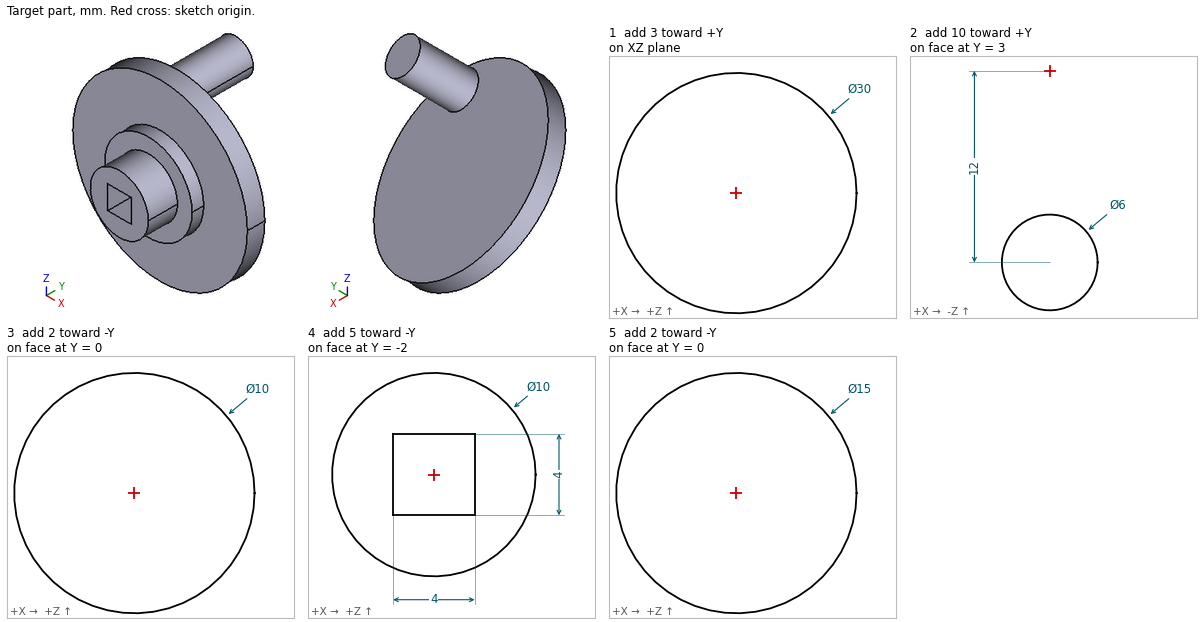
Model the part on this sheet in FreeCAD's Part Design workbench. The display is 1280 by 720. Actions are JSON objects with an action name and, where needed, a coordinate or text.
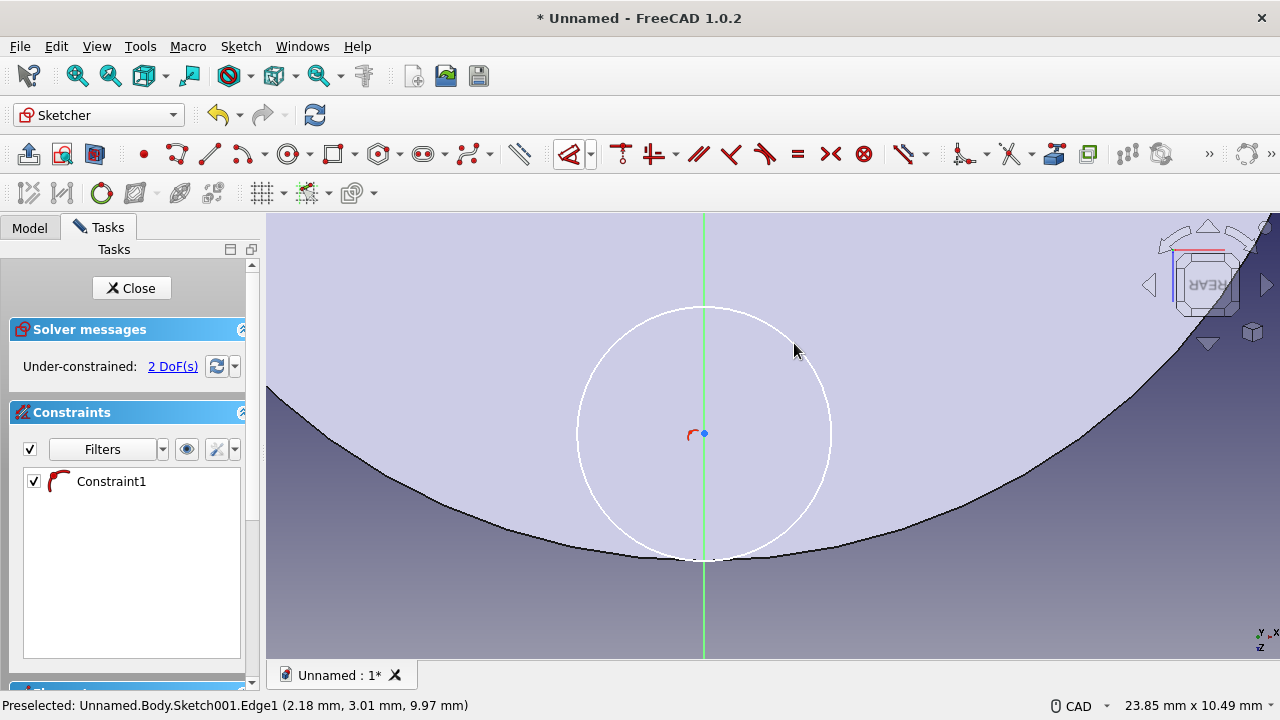
{"action": "left_click", "coordinate": [568, 154]}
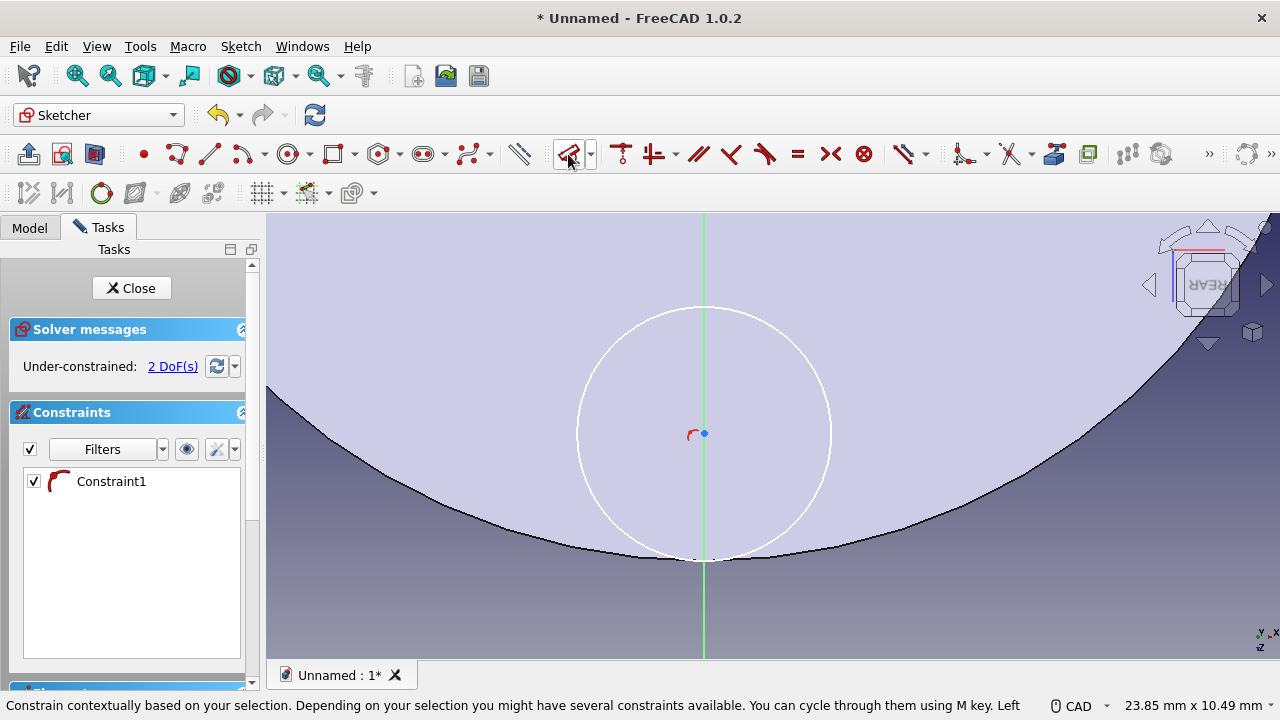
{"action": "left_click", "coordinate": [794, 344]}
{"action": "left_click", "coordinate": [817, 321]}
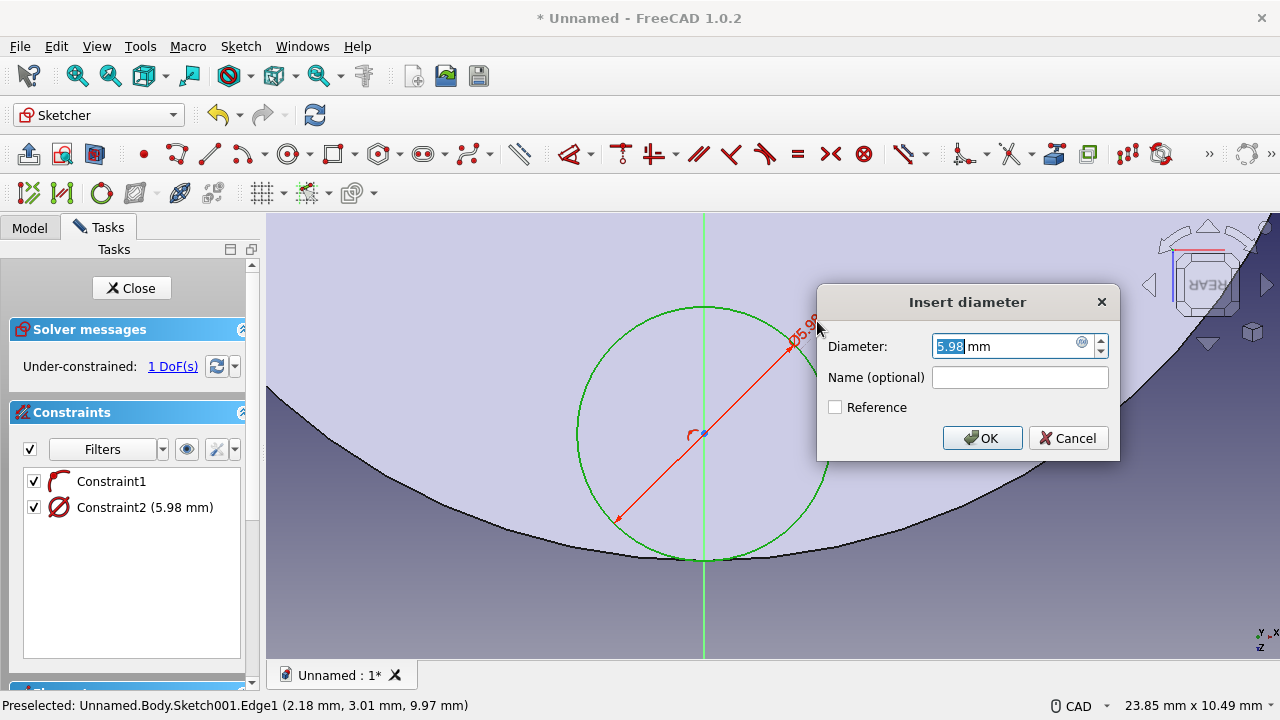
{"action": "type", "text": "6"}
{"action": "key", "text": "Return"}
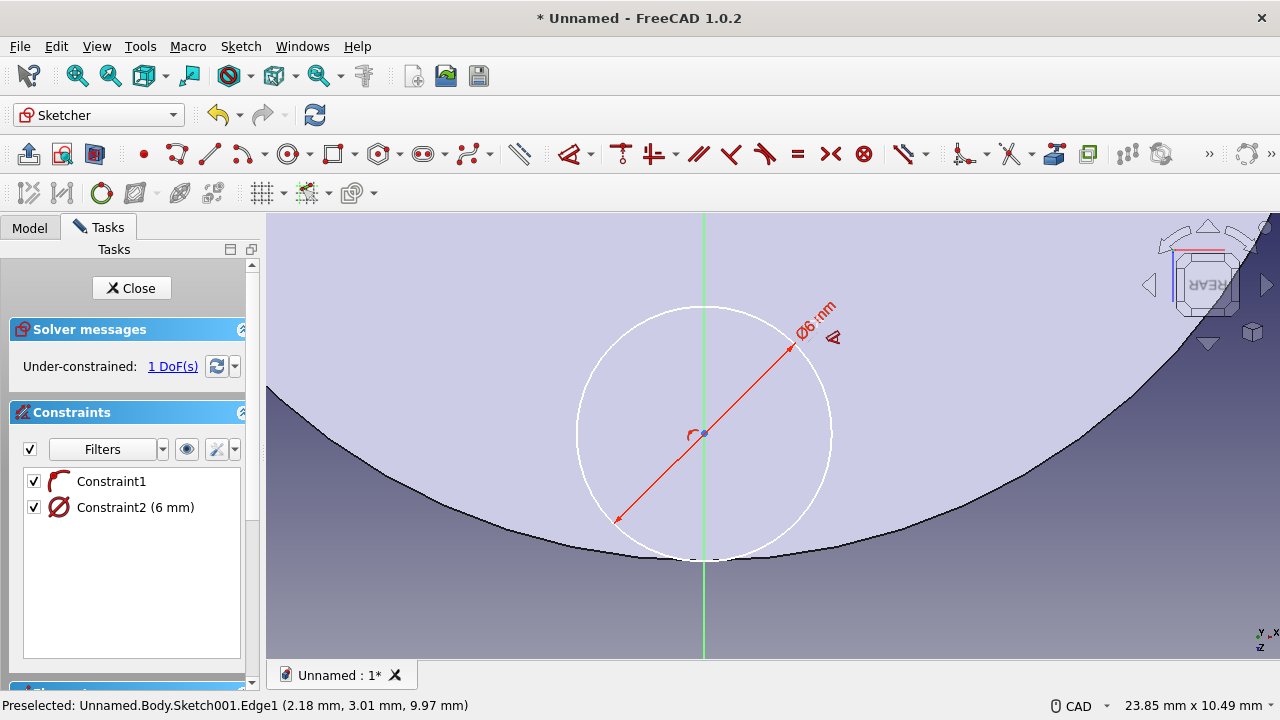
{"action": "left_click", "coordinate": [704, 434]}
{"action": "left_click", "coordinate": [738, 337]}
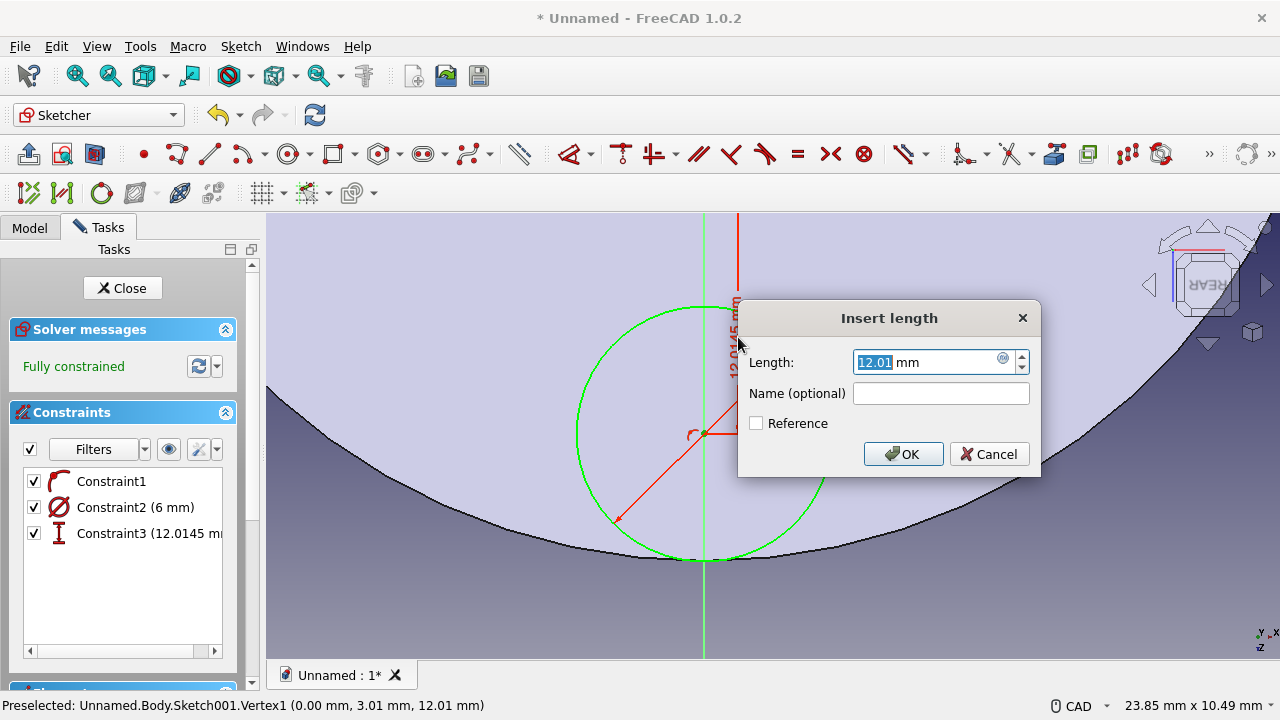
{"action": "type", "text": "12"}
{"action": "key", "text": "Return"}
{"action": "key", "text": "Escape"}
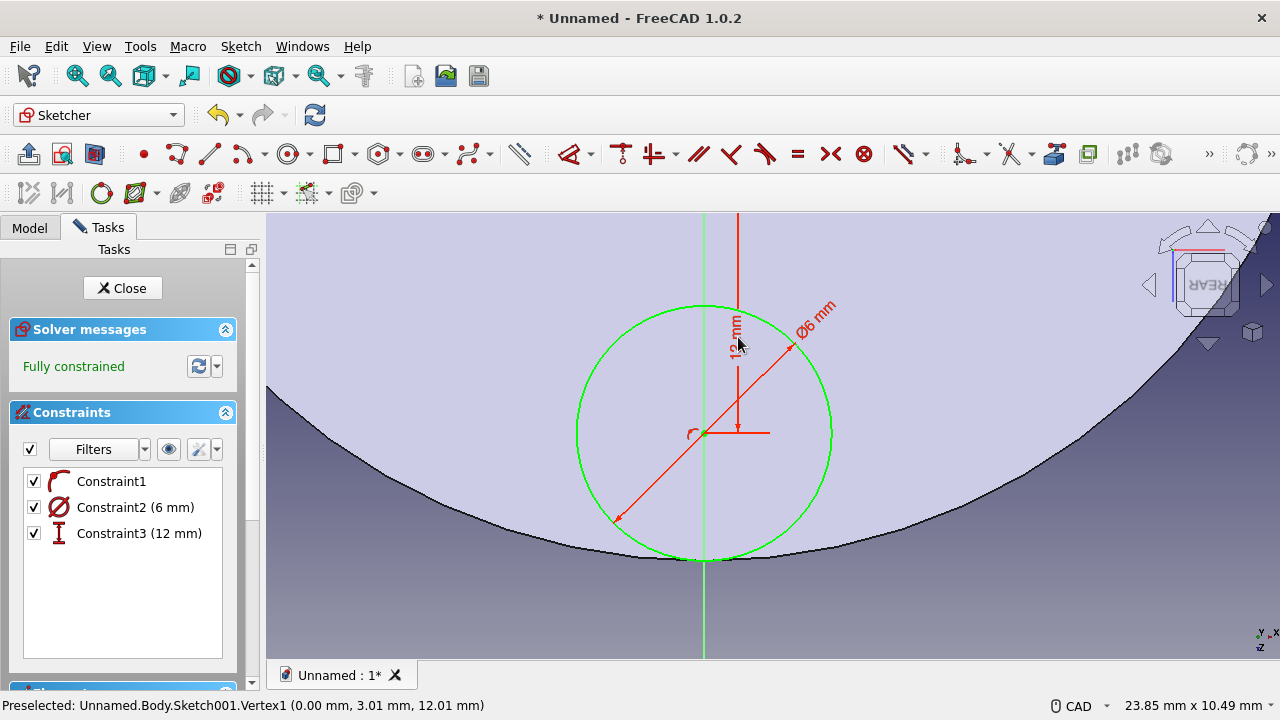
{"action": "left_click", "coordinate": [123, 288]}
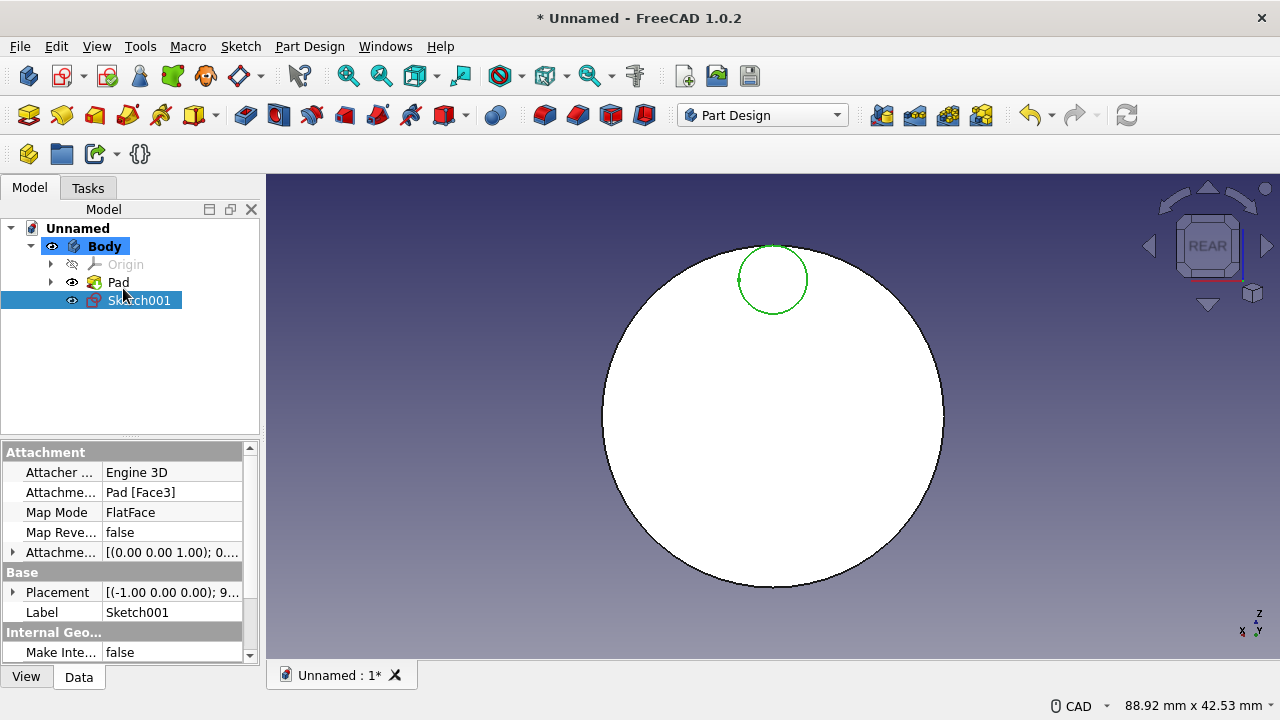
{"action": "left_click", "coordinate": [29, 116]}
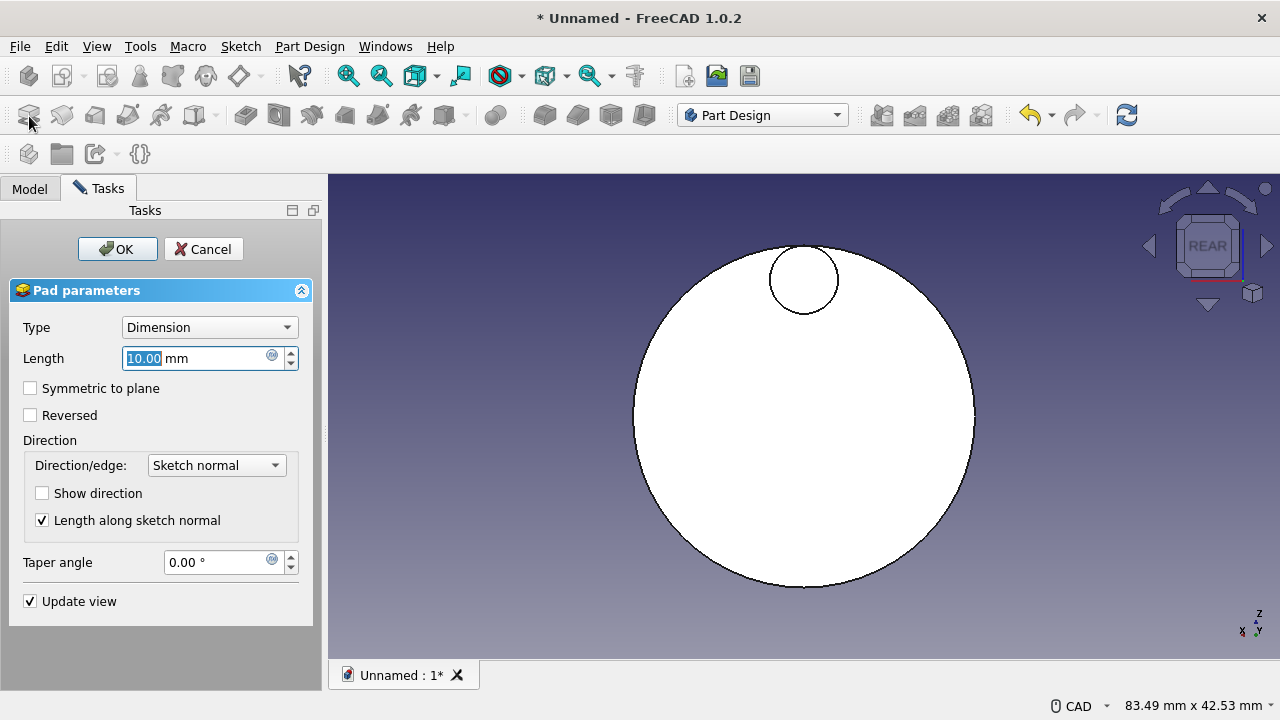
{"action": "type", "text": "10"}
{"action": "key", "text": "Tab"}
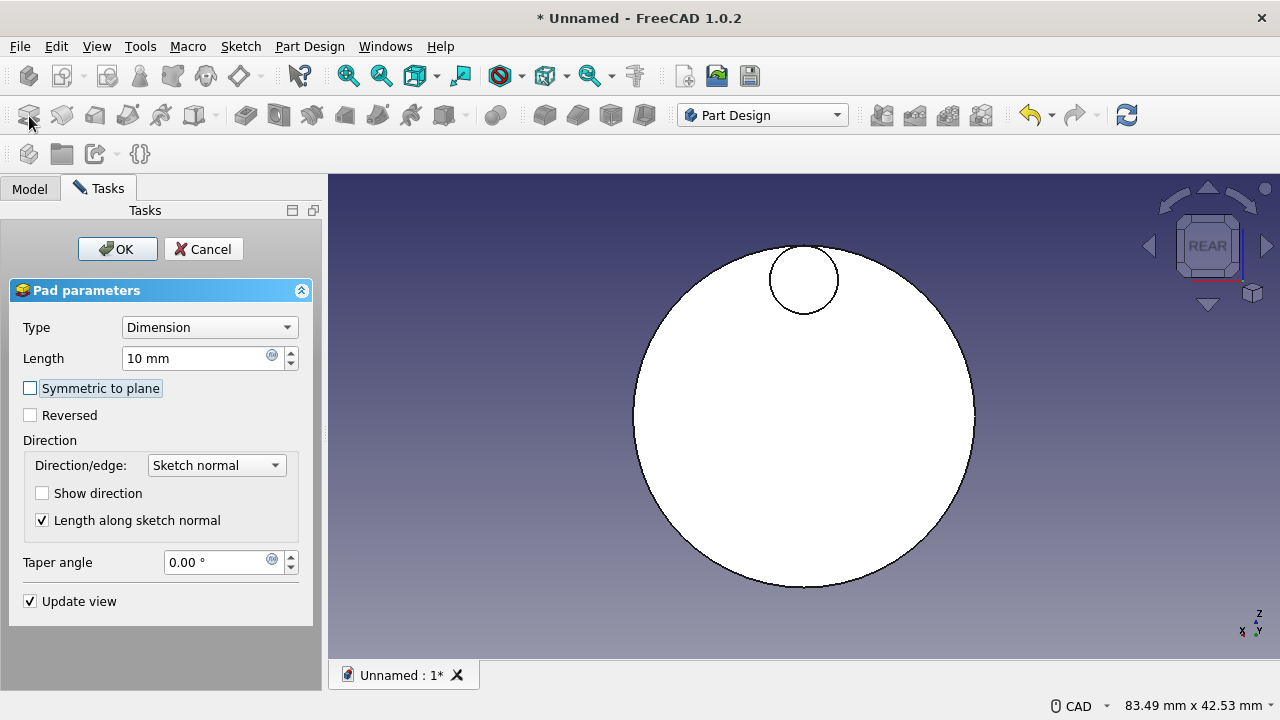
{"action": "left_click", "coordinate": [118, 249]}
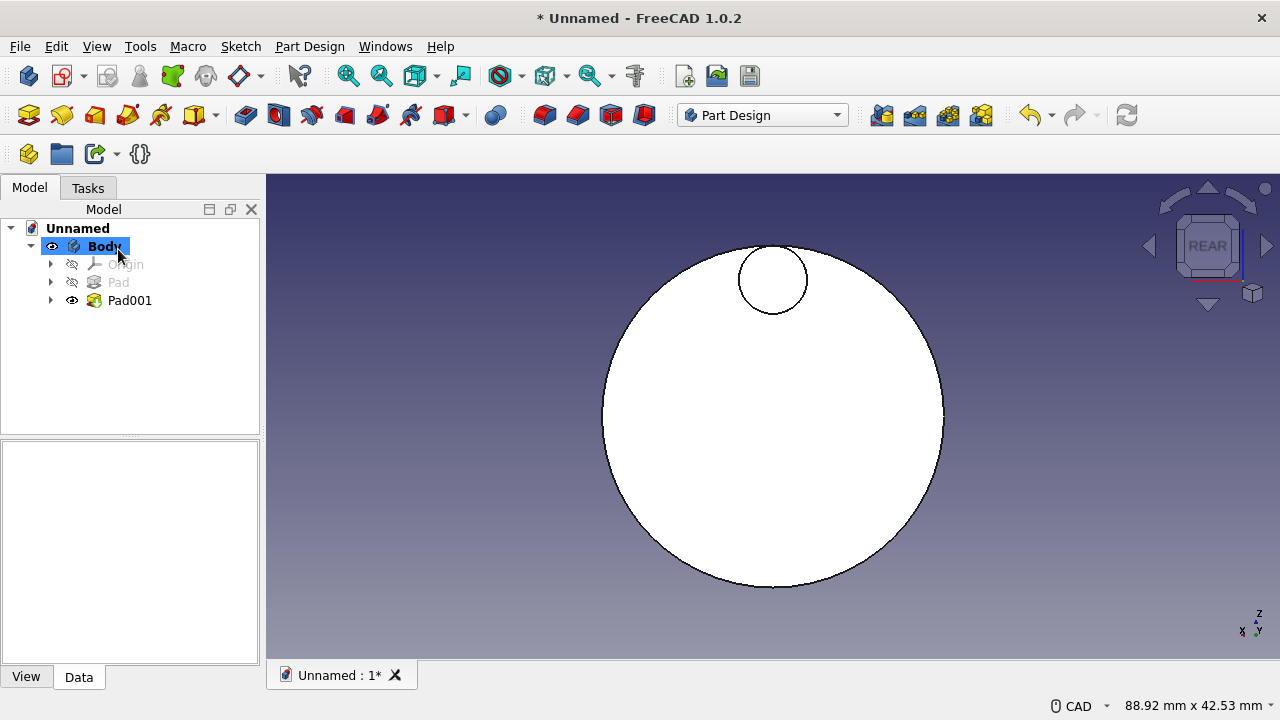
{"action": "key", "text": "0"}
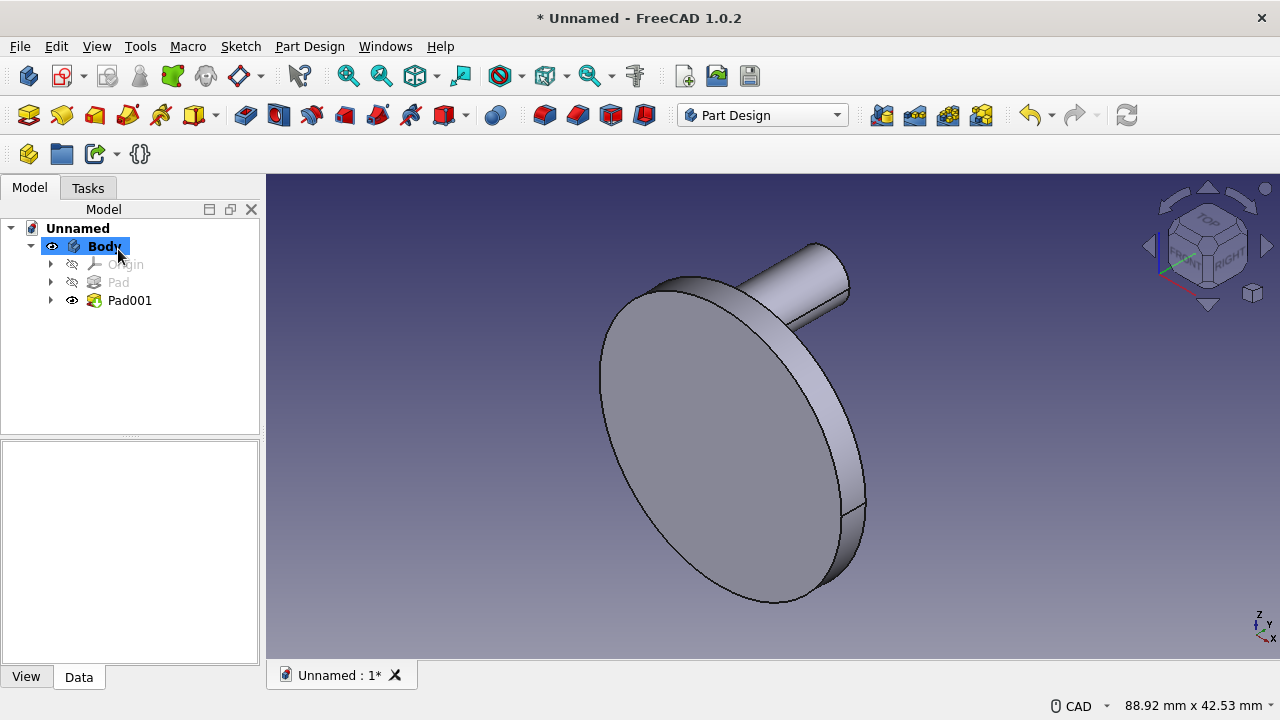
{"action": "left_click", "coordinate": [721, 446]}